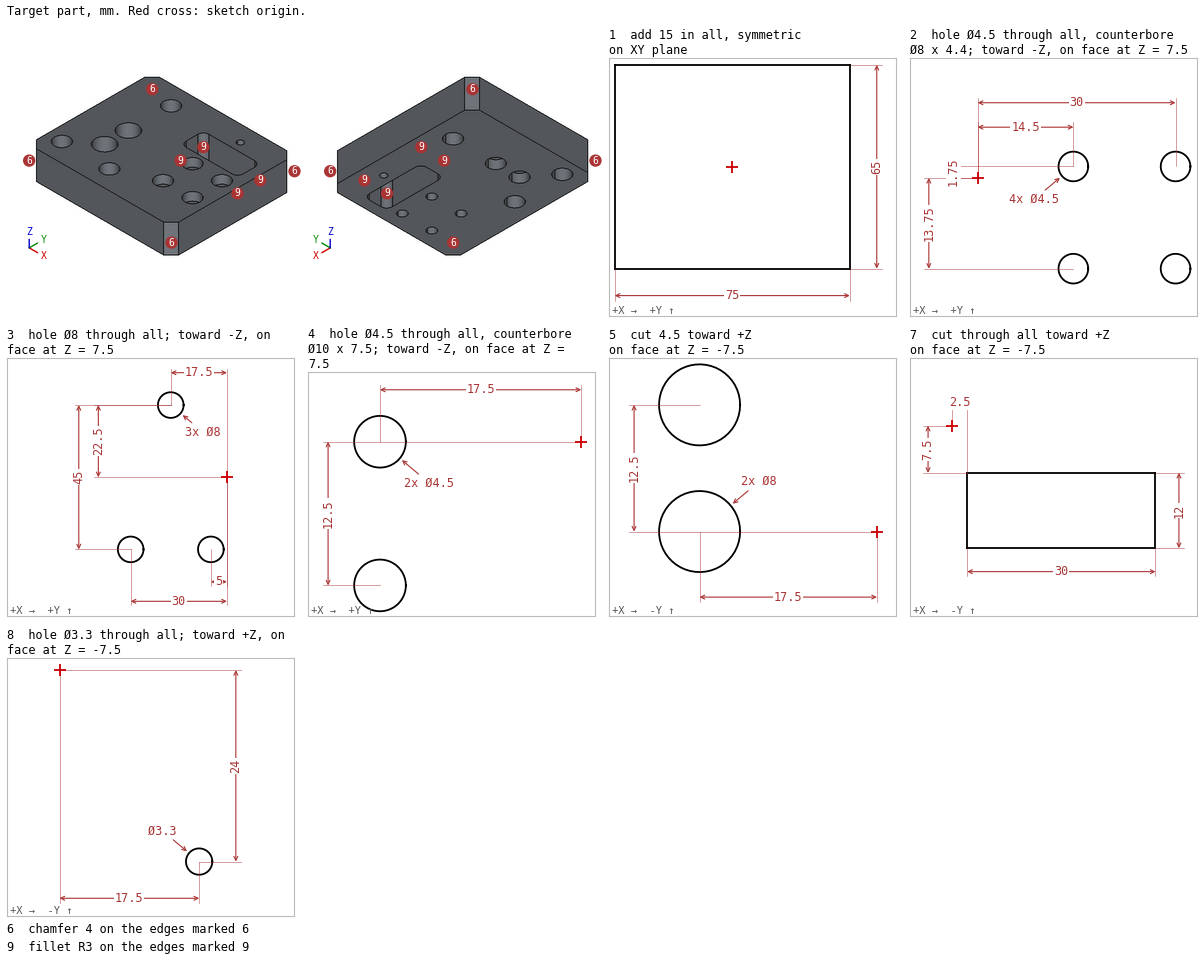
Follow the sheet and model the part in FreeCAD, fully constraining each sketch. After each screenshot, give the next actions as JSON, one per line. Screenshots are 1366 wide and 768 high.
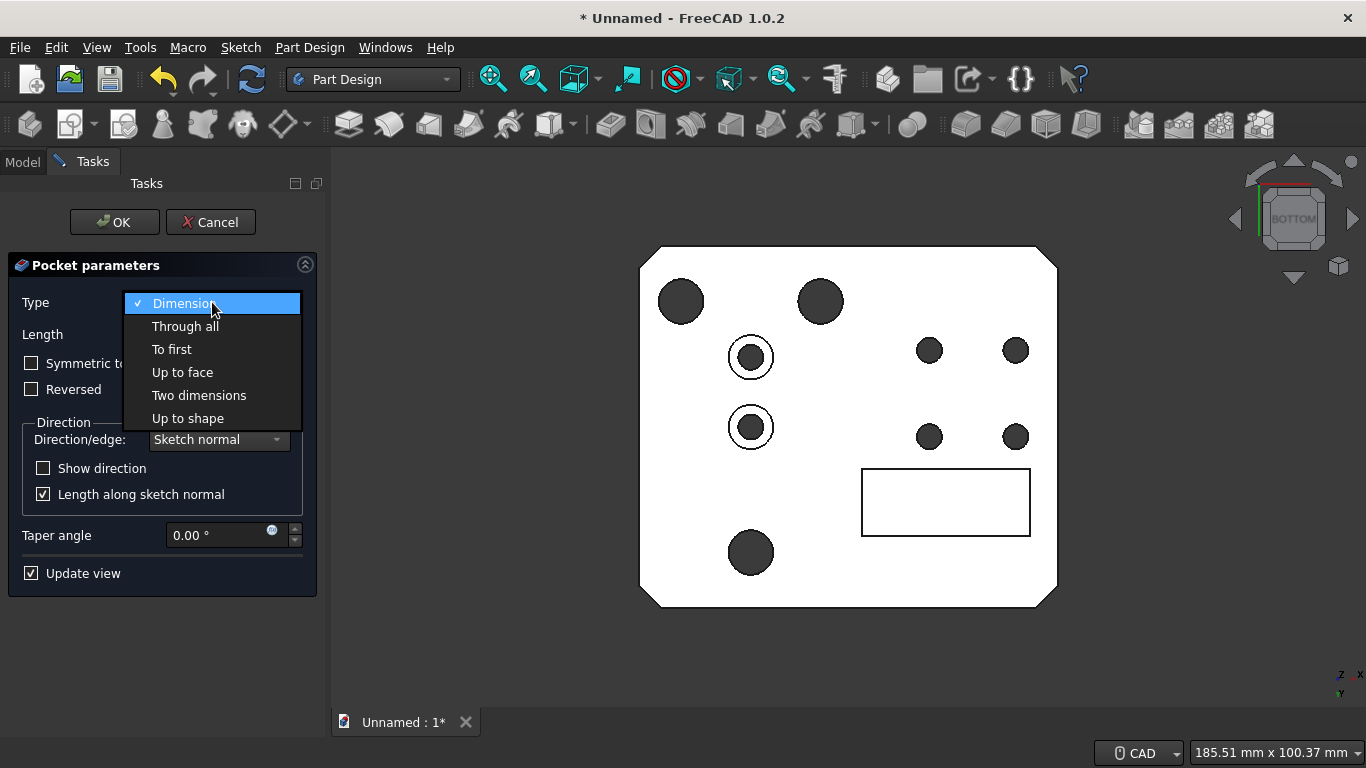
{"action": "left_click", "coordinate": [212, 326]}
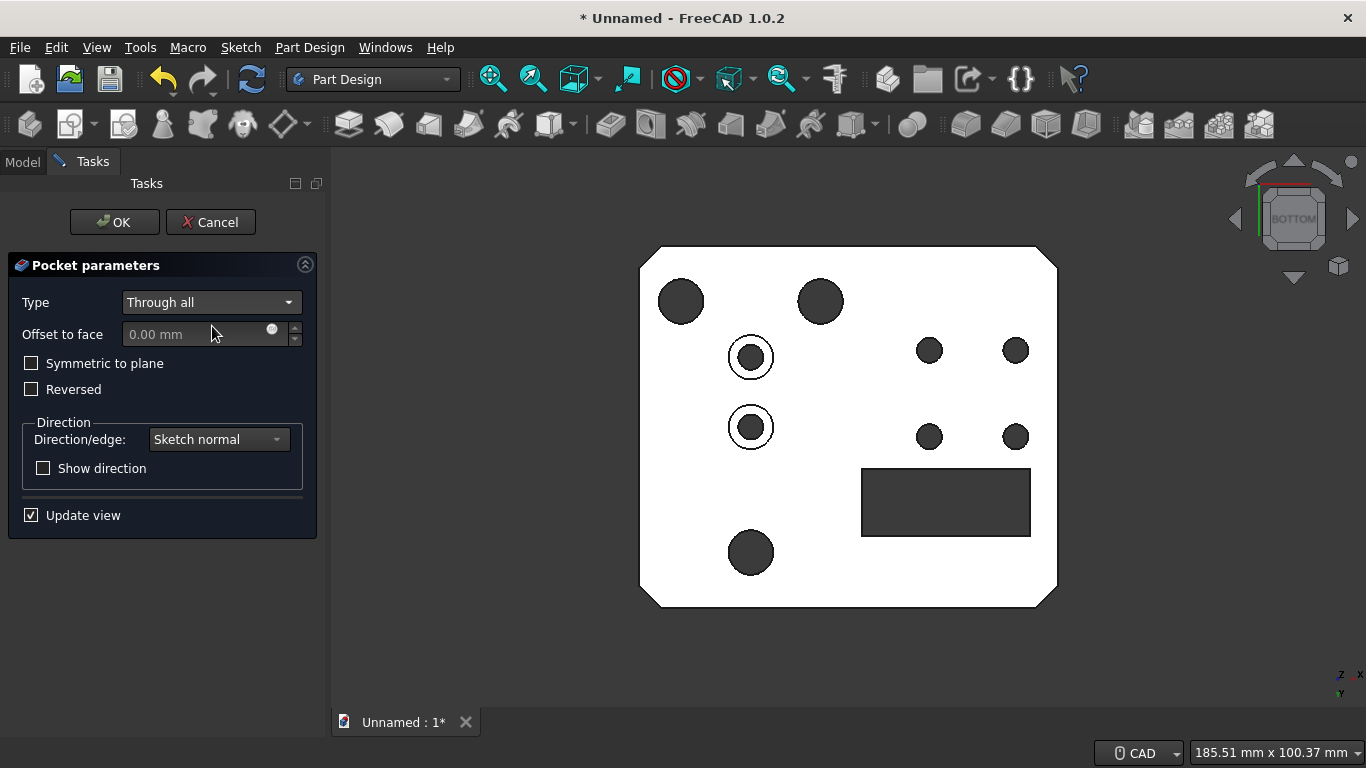
{"action": "left_click", "coordinate": [115, 222]}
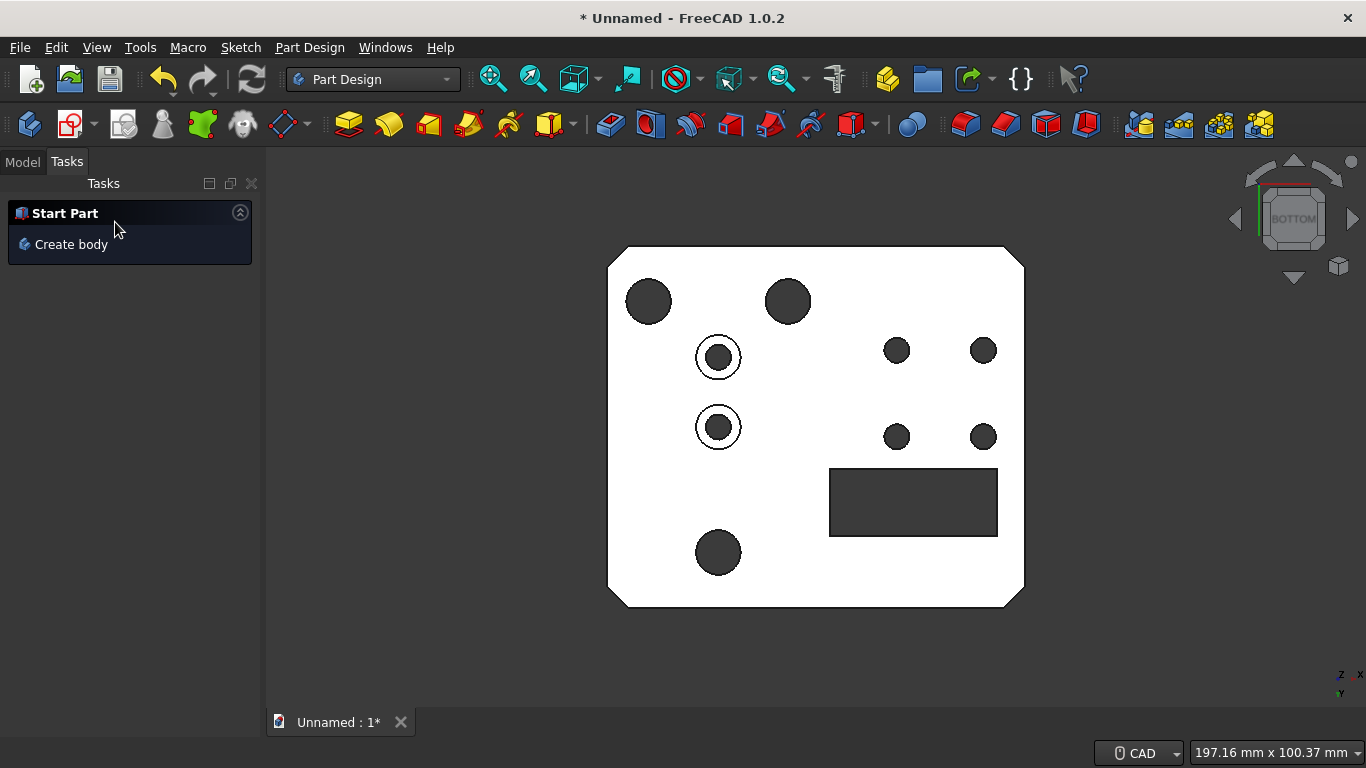
{"action": "left_click", "coordinate": [816, 374]}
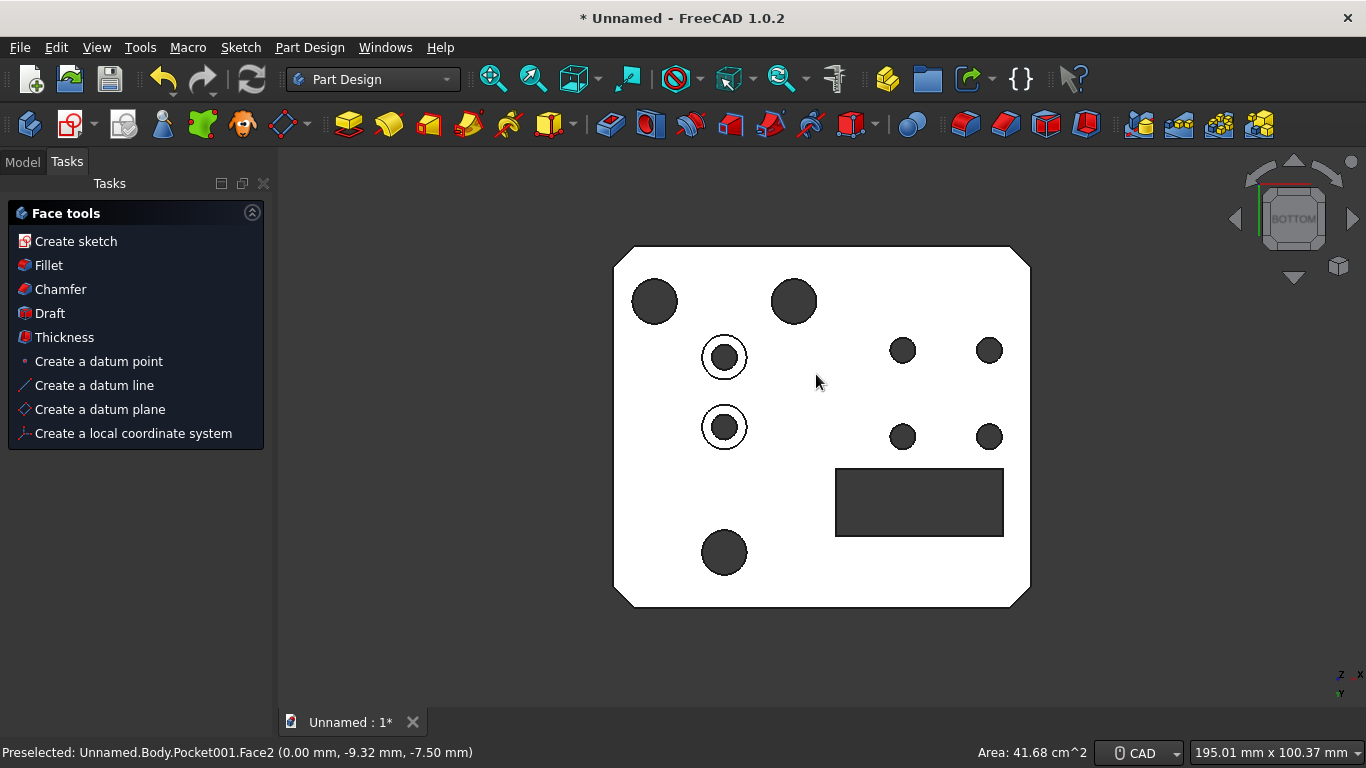
{"action": "left_click", "coordinate": [70, 124]}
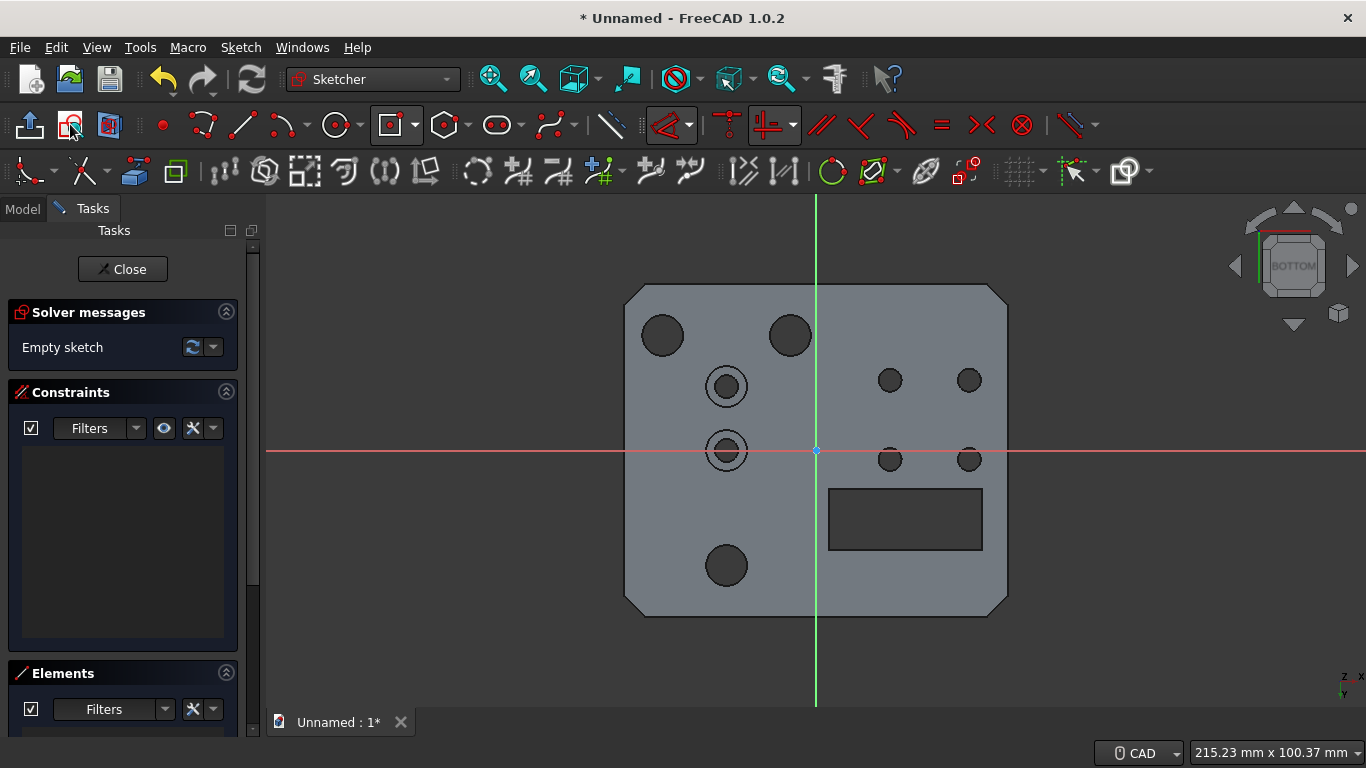
{"action": "scroll", "coordinate": [914, 580], "scroll_direction": "up", "scroll_amount": 15}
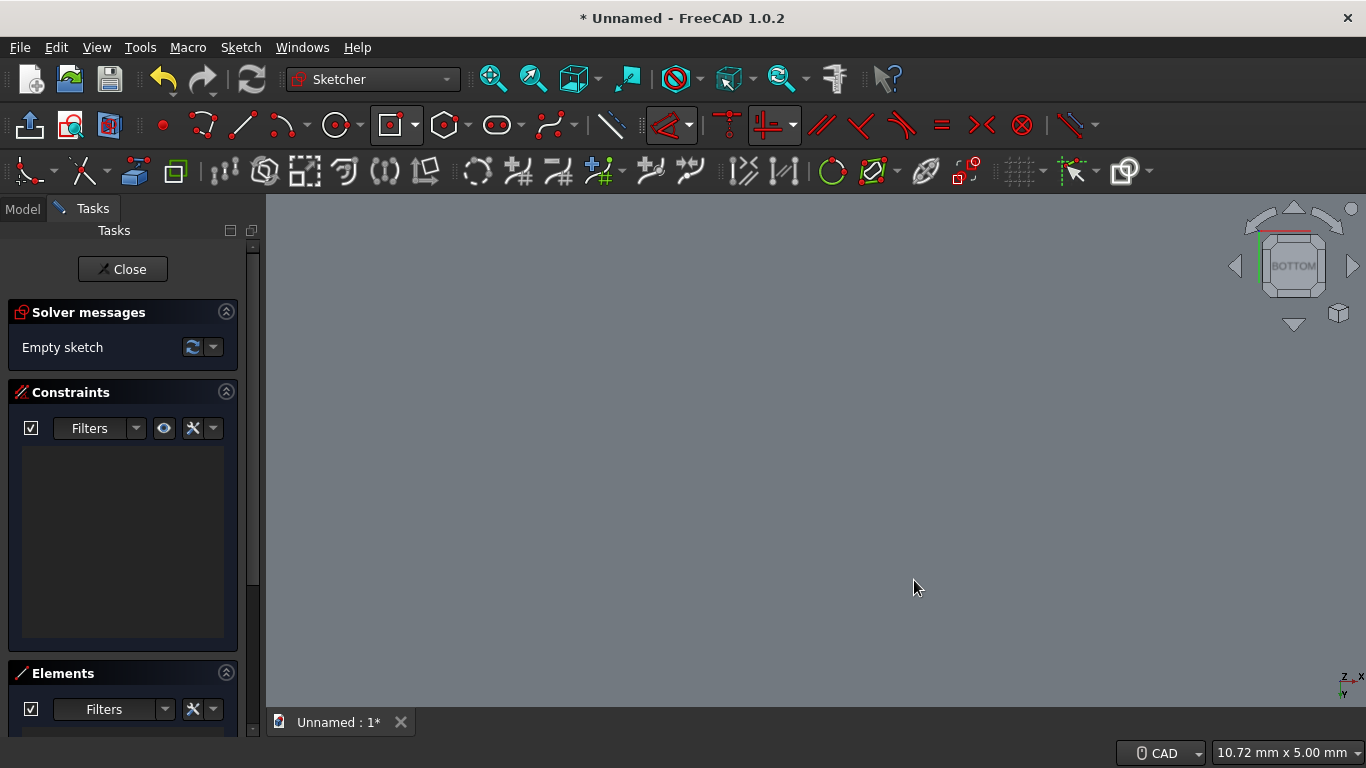
{"action": "key", "text": "g c"}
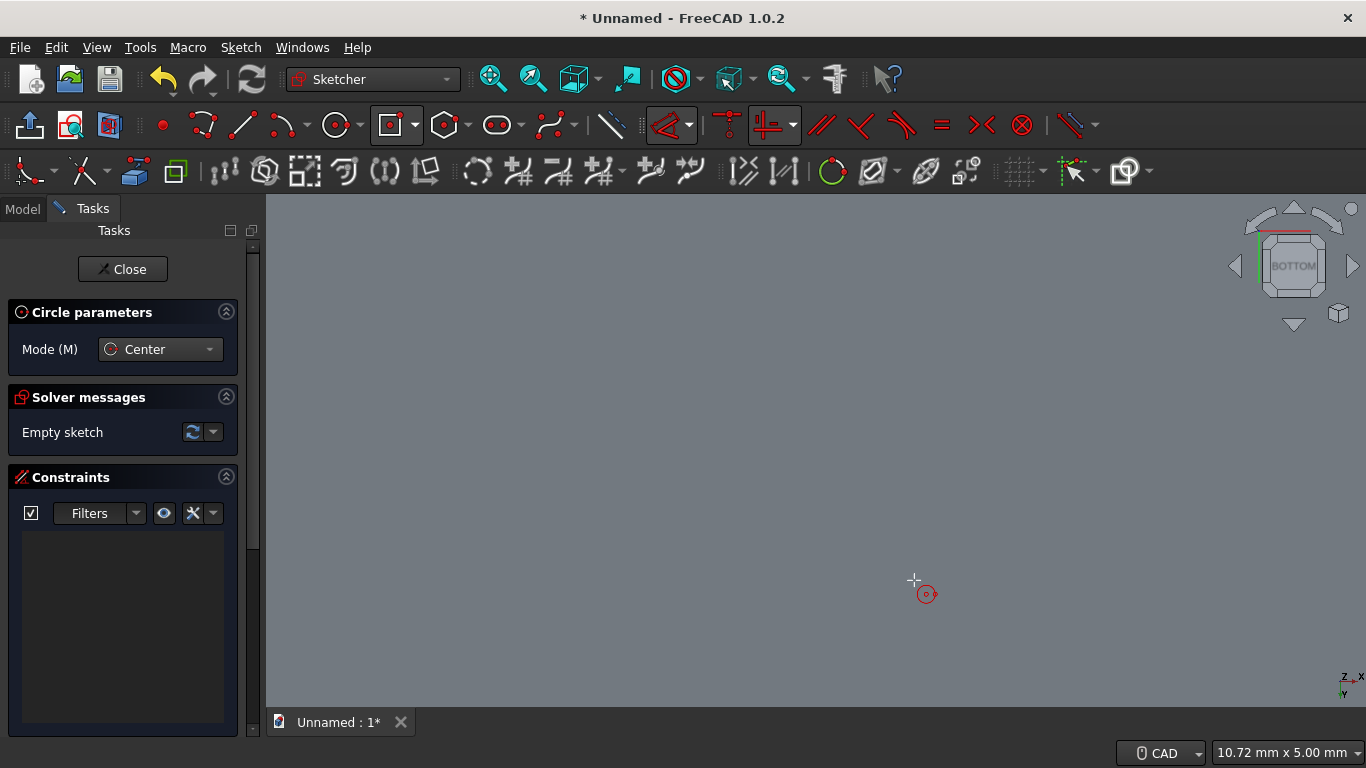
{"action": "left_click", "coordinate": [731, 428]}
{"action": "mouse_move", "coordinate": [851, 308]}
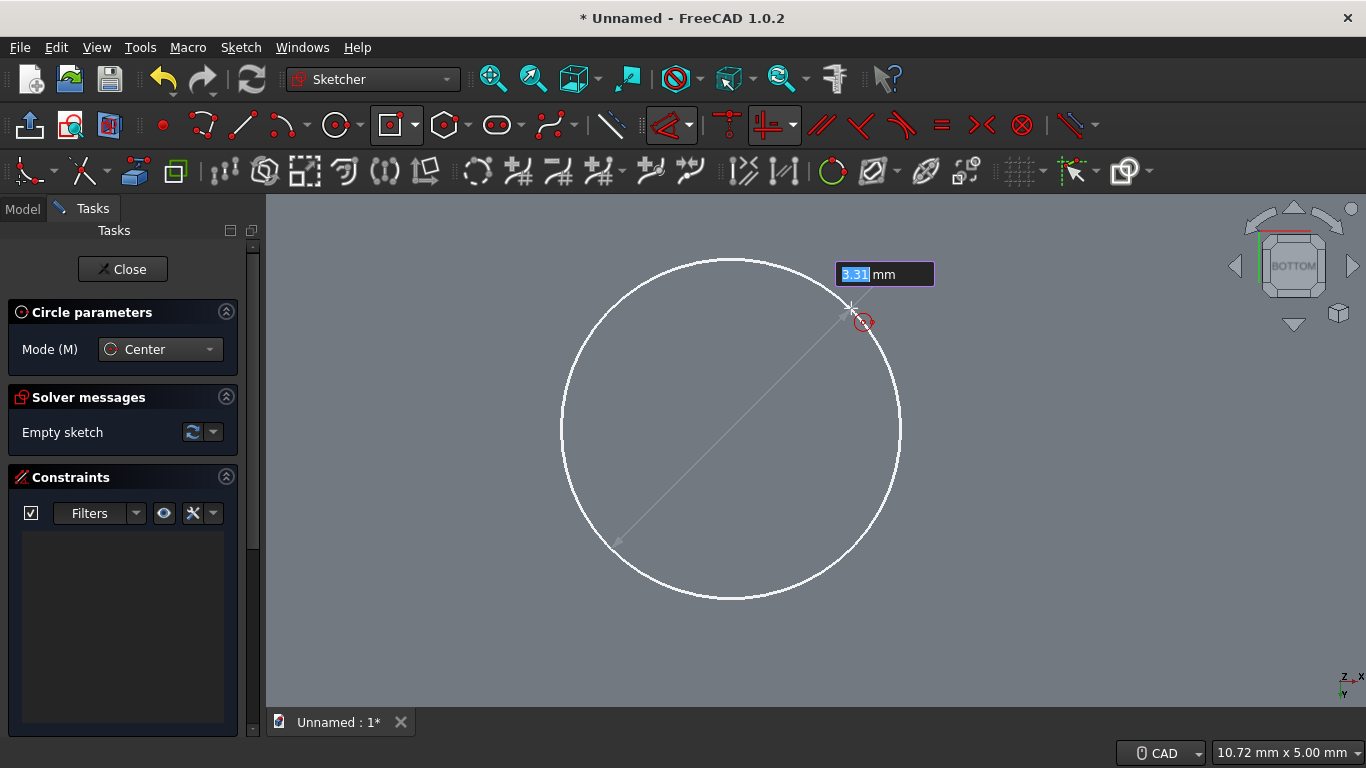
{"action": "type", "text": "3.3"}
{"action": "key", "text": "Return"}
{"action": "key", "text": "Escape"}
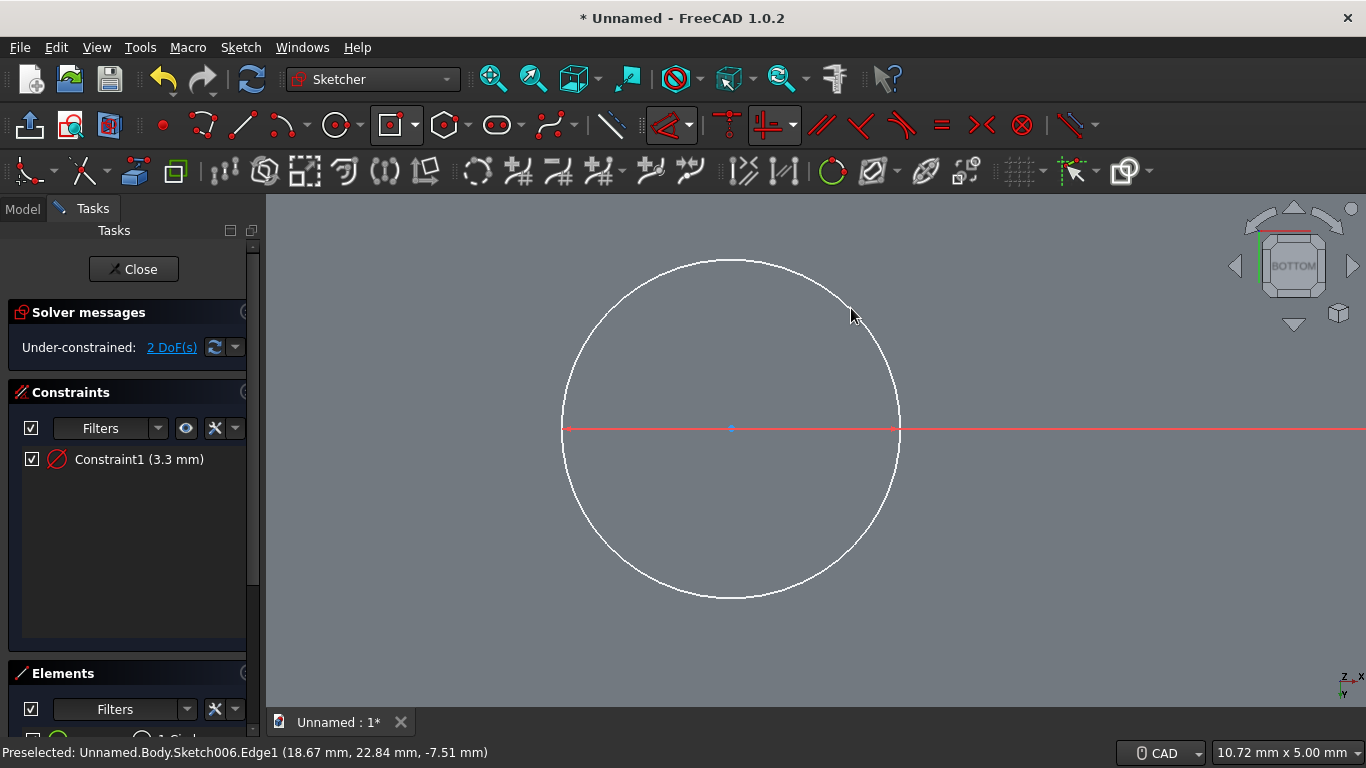
{"action": "left_click", "coordinate": [731, 429]}